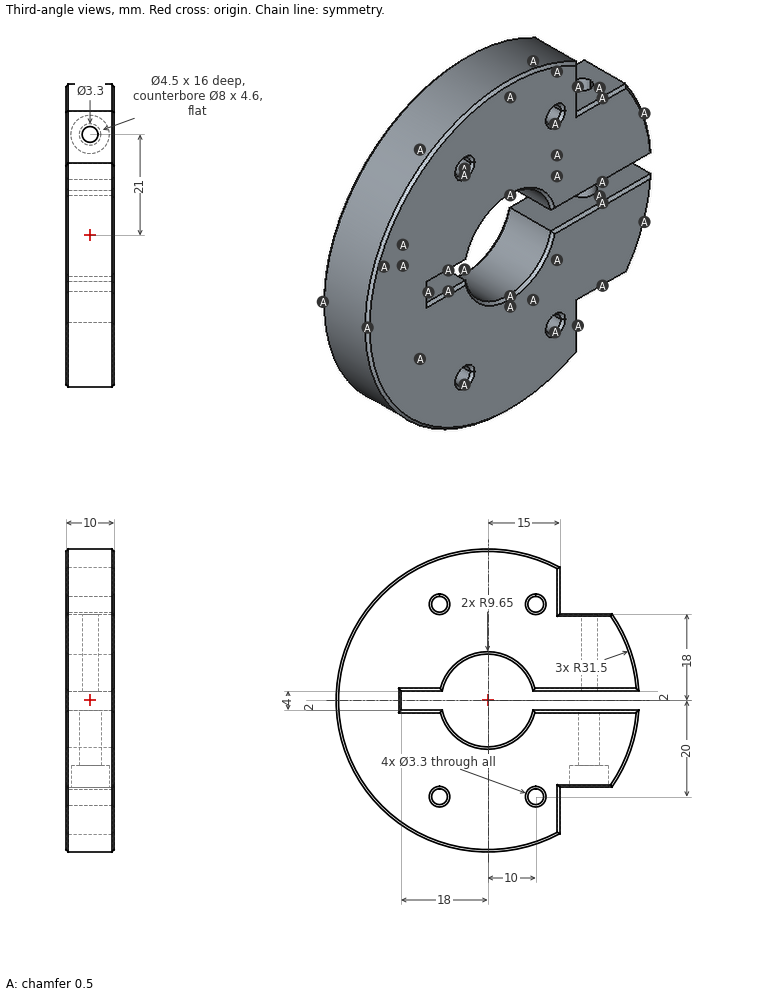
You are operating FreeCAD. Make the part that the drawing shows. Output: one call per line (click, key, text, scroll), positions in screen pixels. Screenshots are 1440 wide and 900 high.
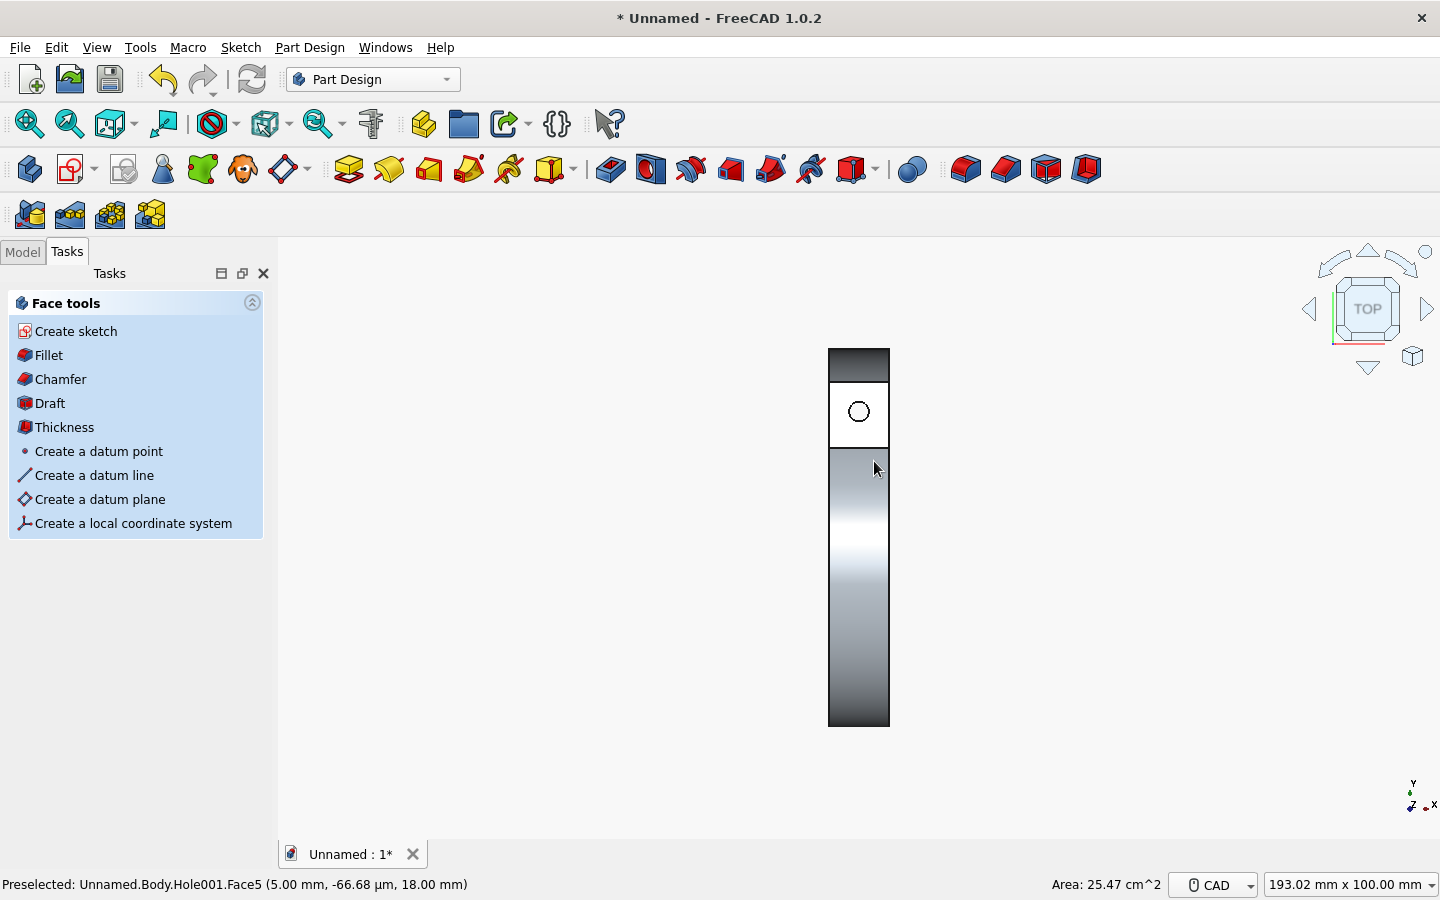
key(0)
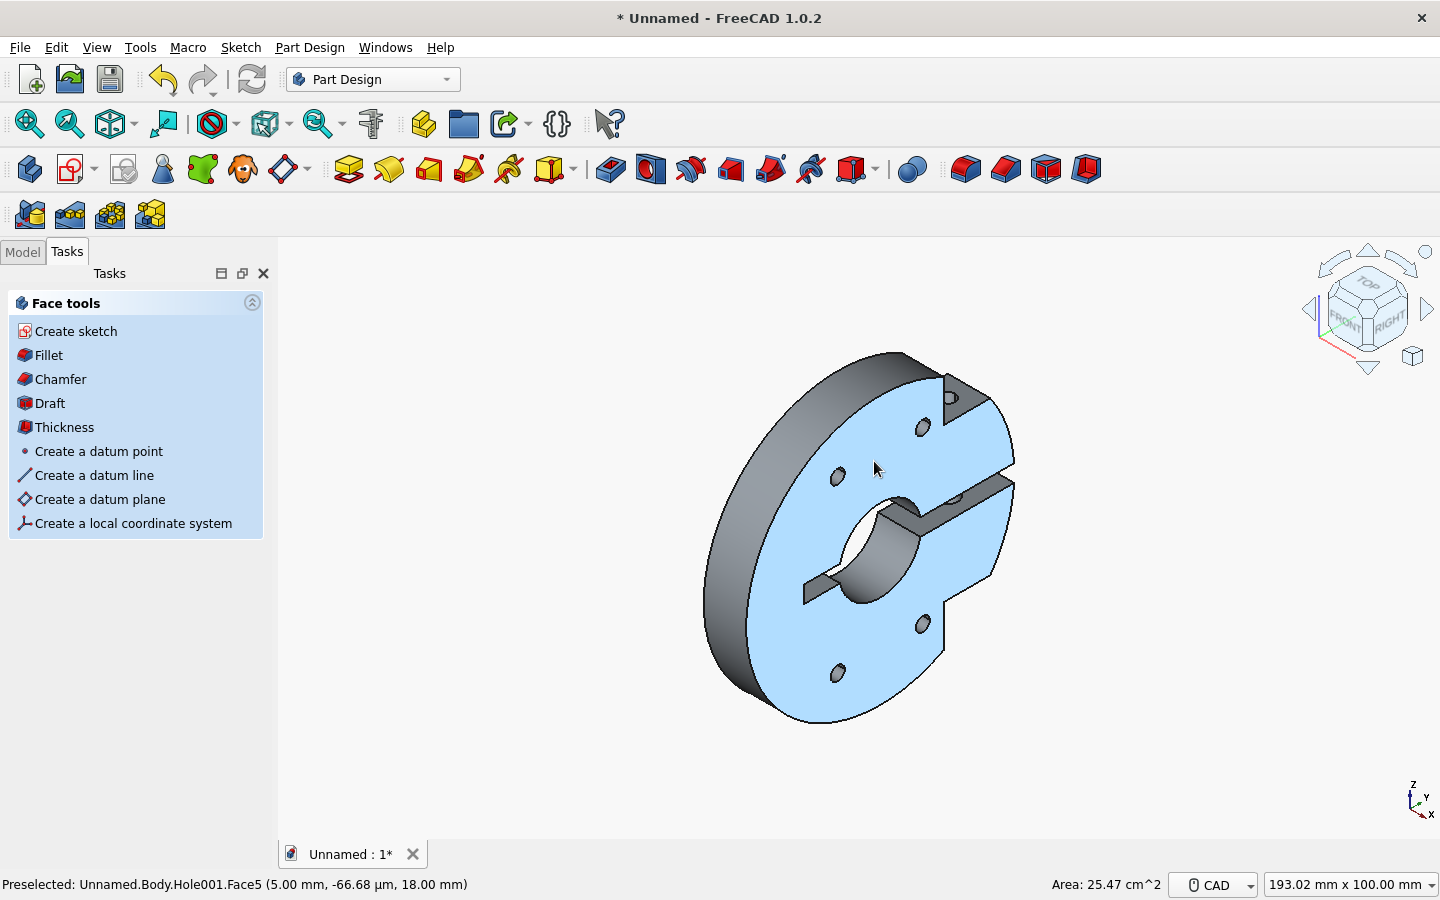
key(1)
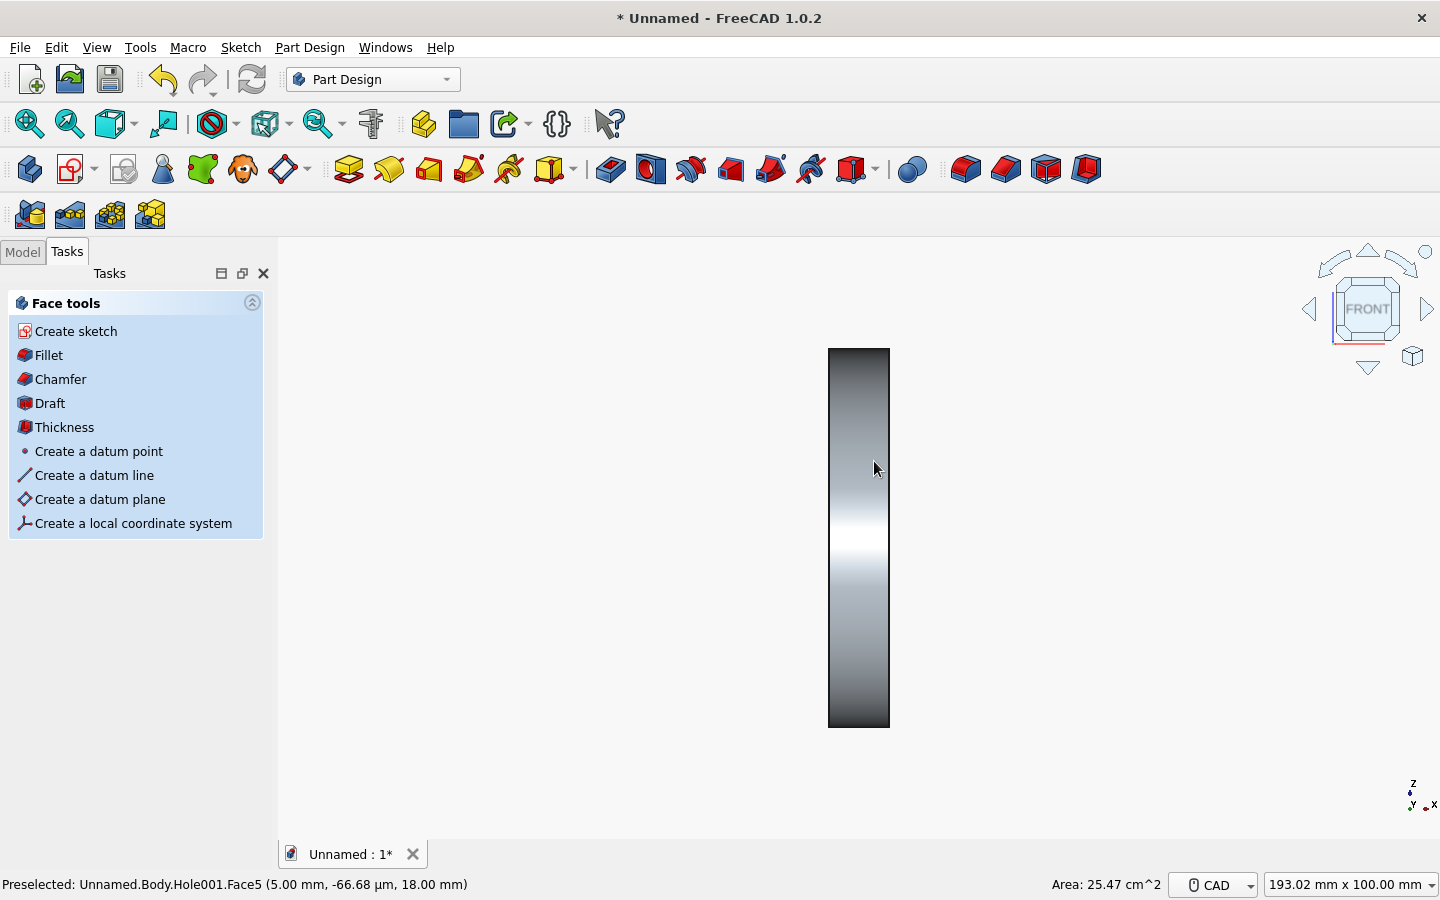
key(3)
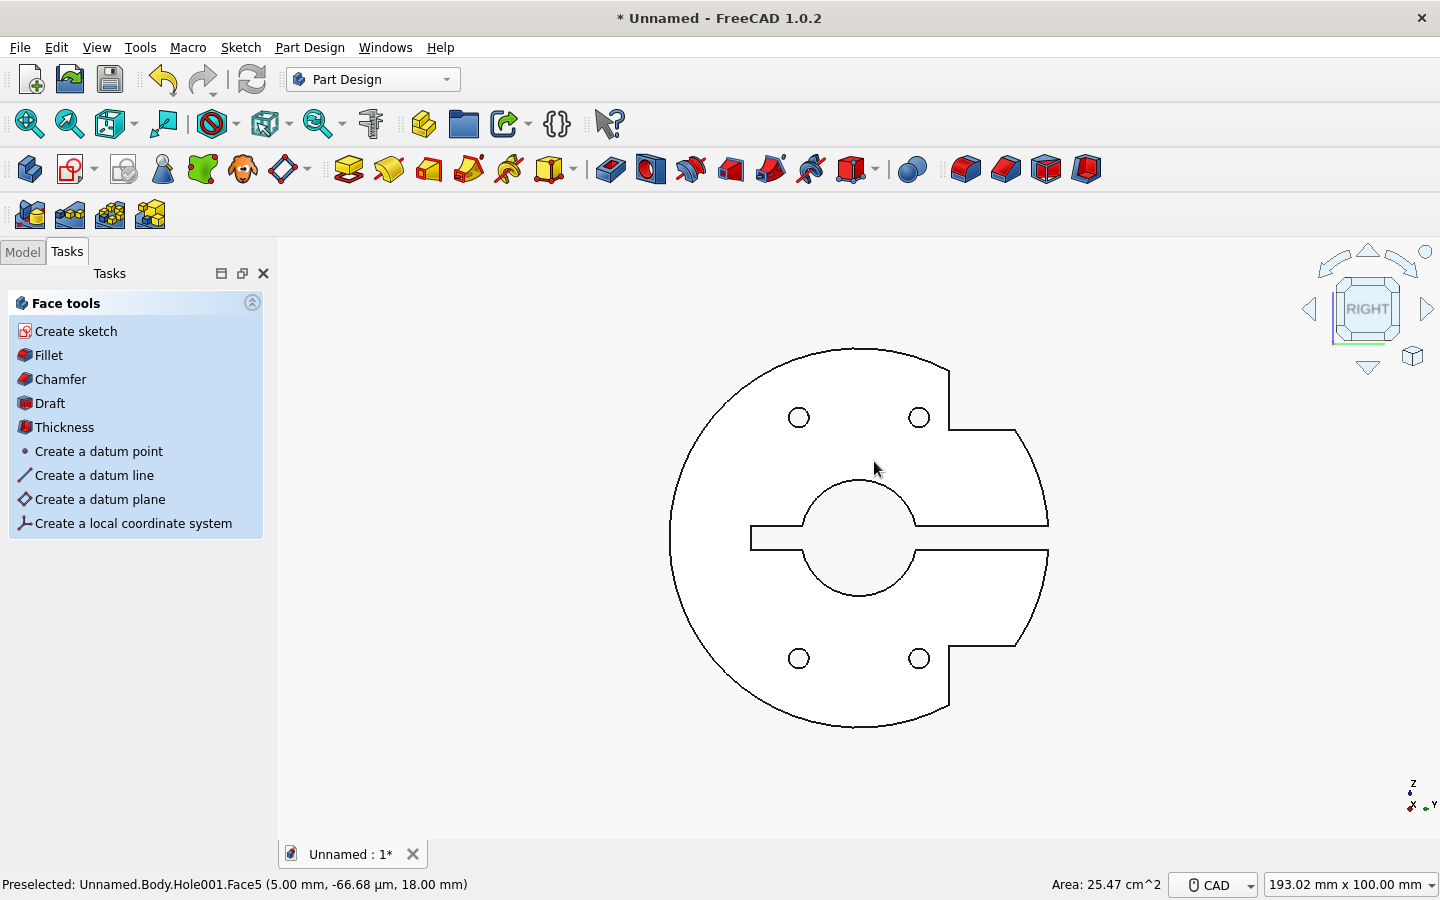
key(5)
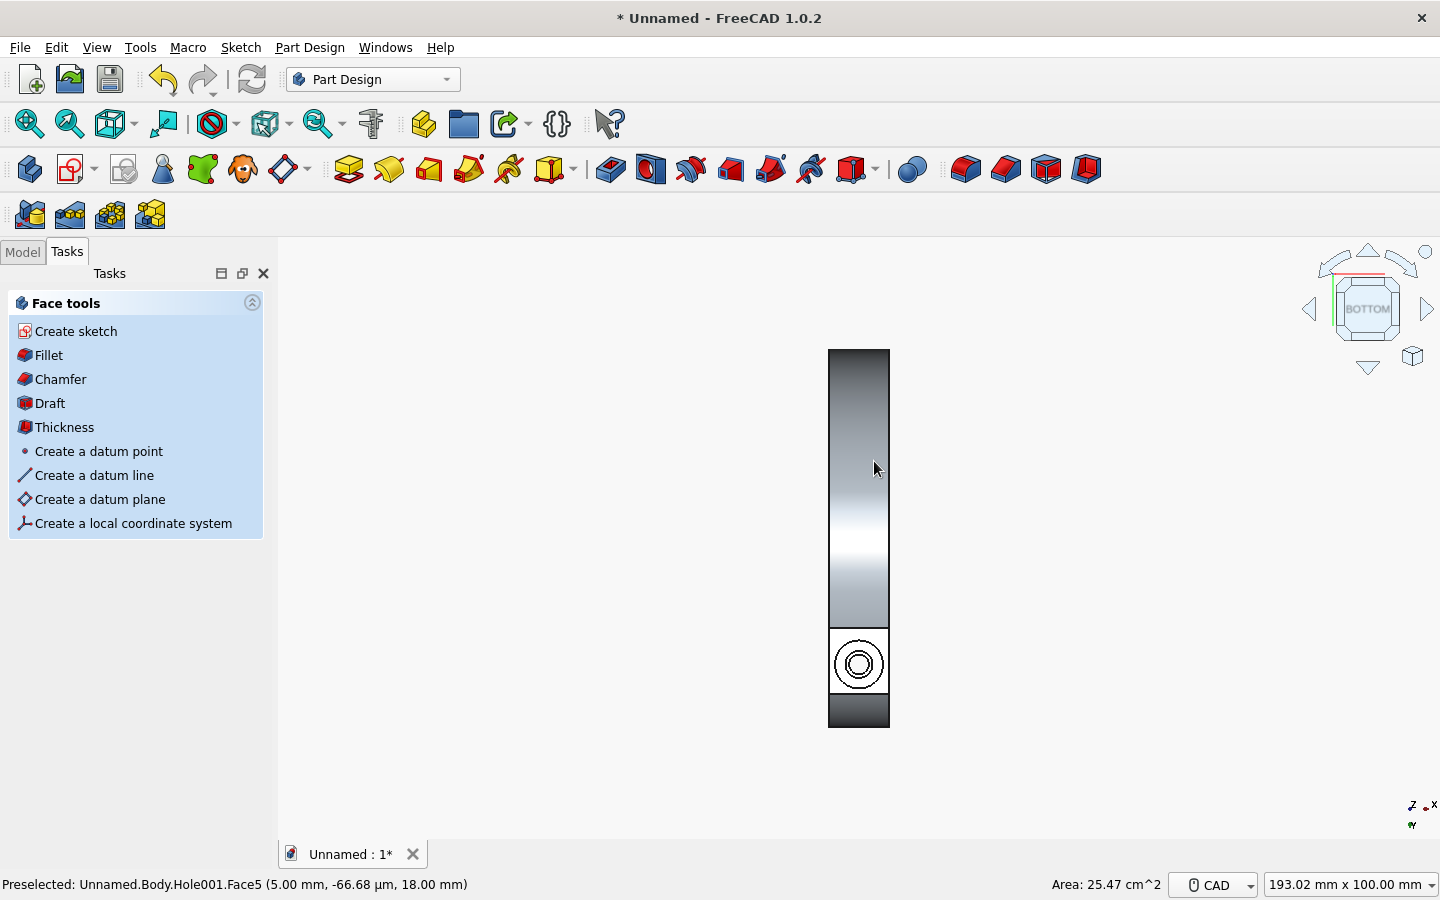
key(4)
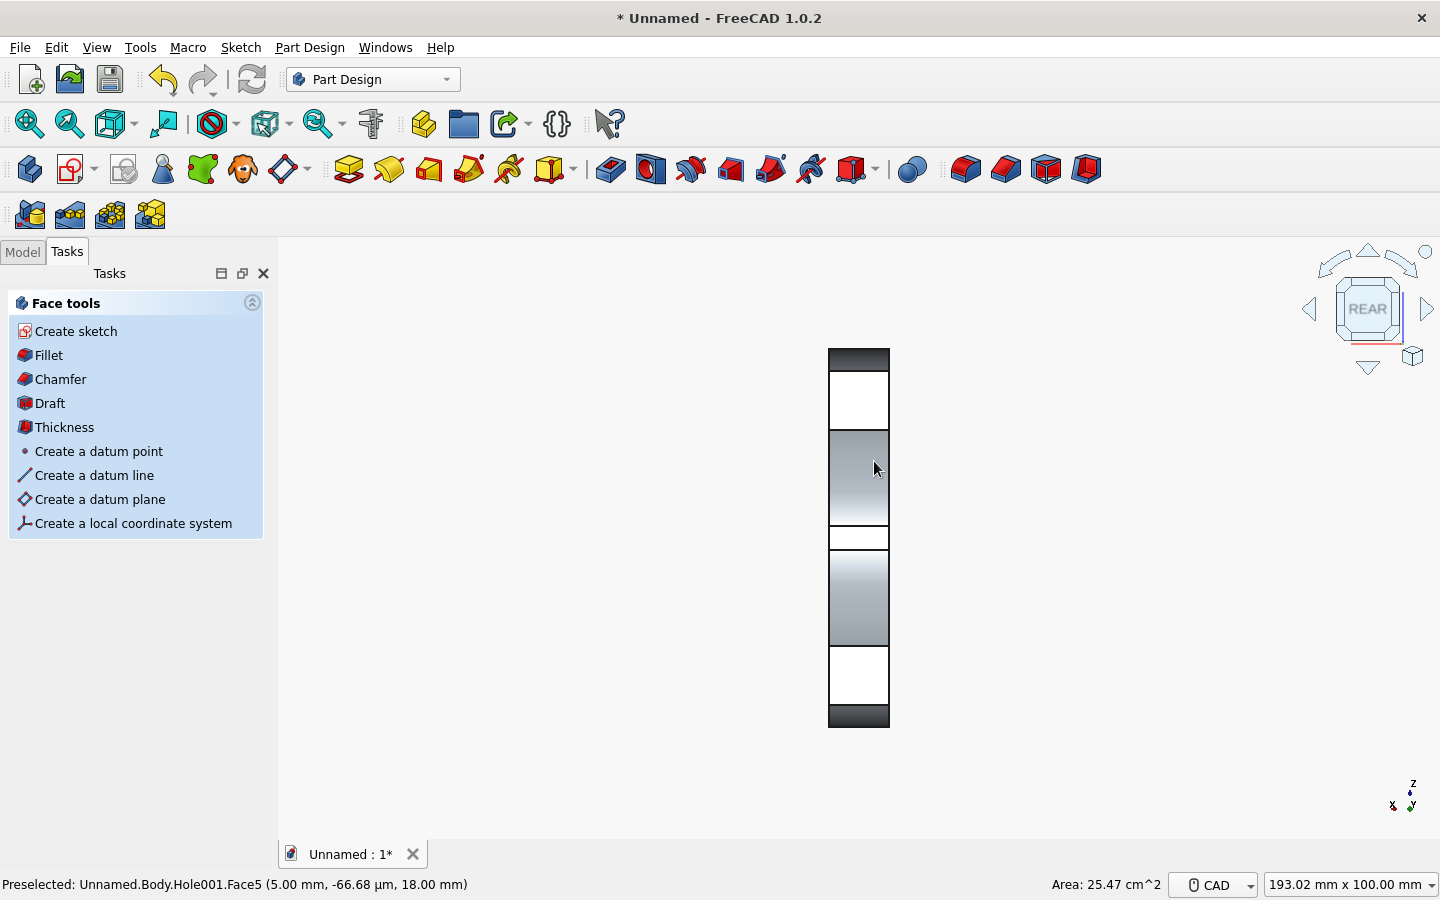
key(6)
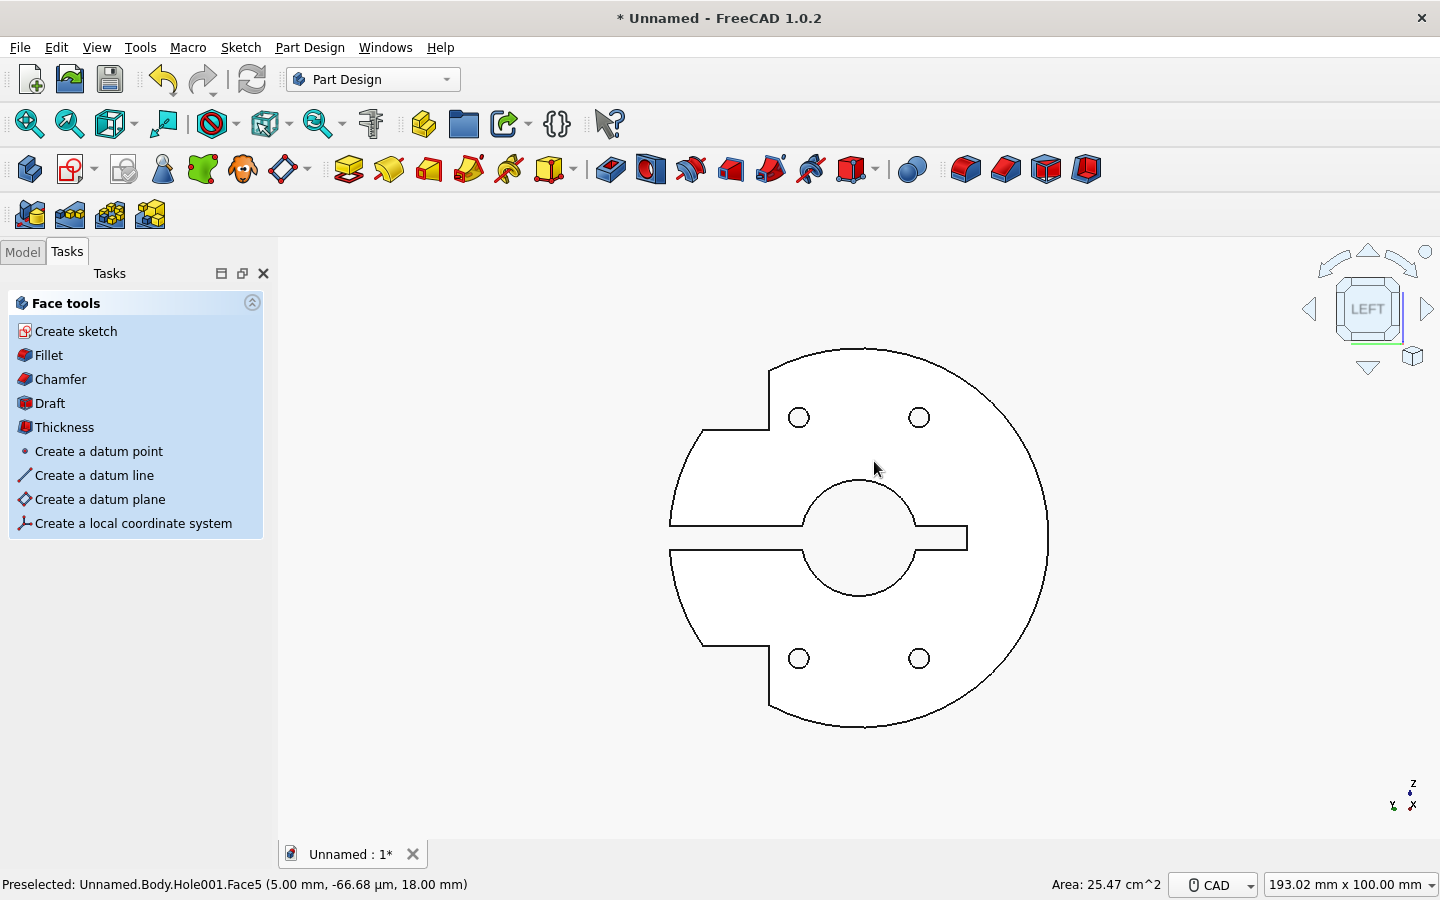
click(859, 645, ctrl)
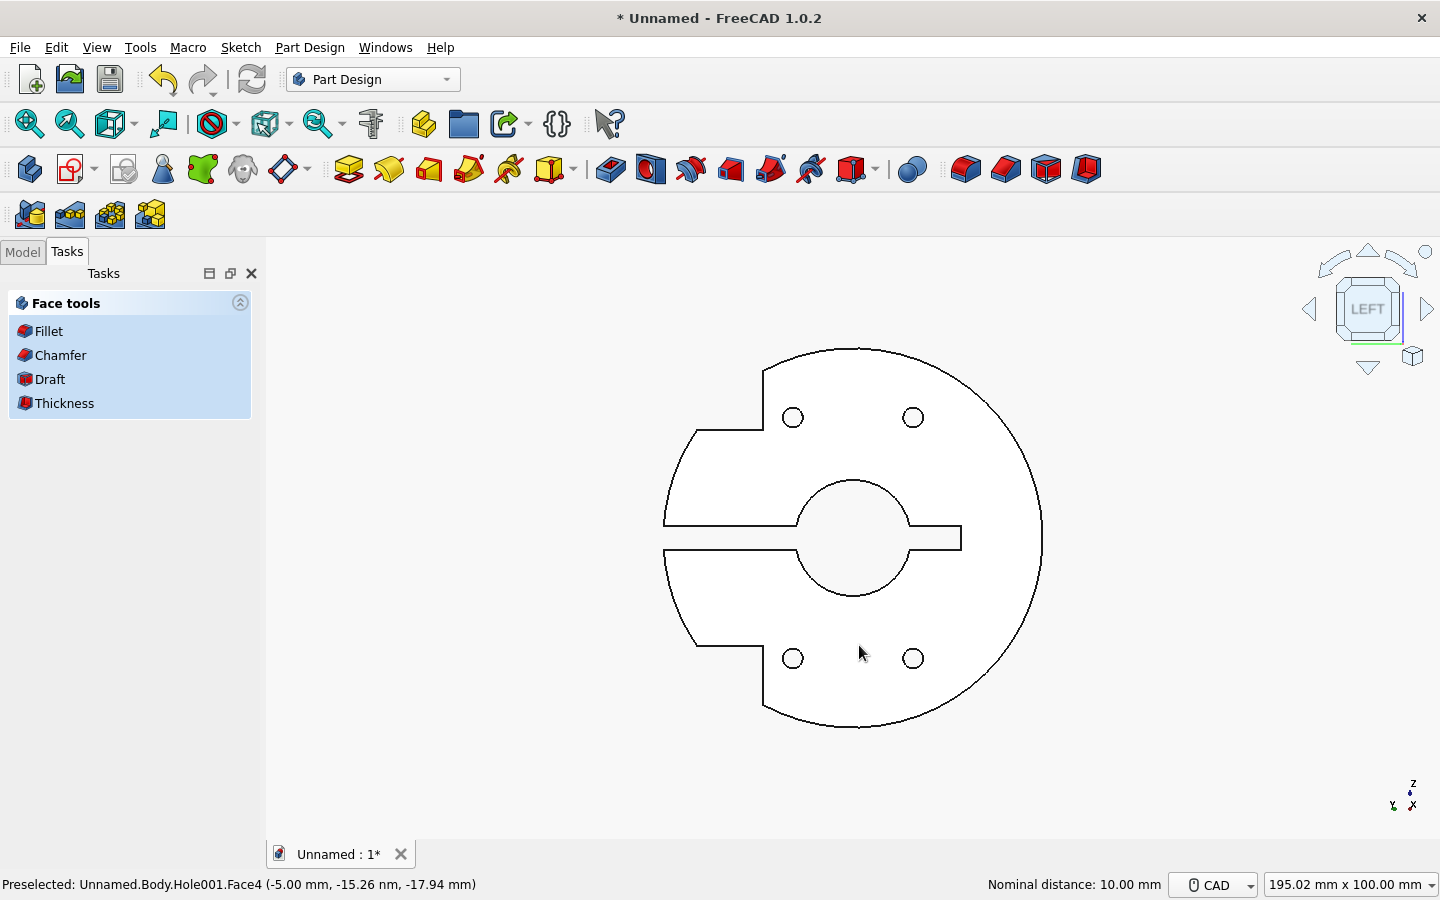
click(1006, 170)